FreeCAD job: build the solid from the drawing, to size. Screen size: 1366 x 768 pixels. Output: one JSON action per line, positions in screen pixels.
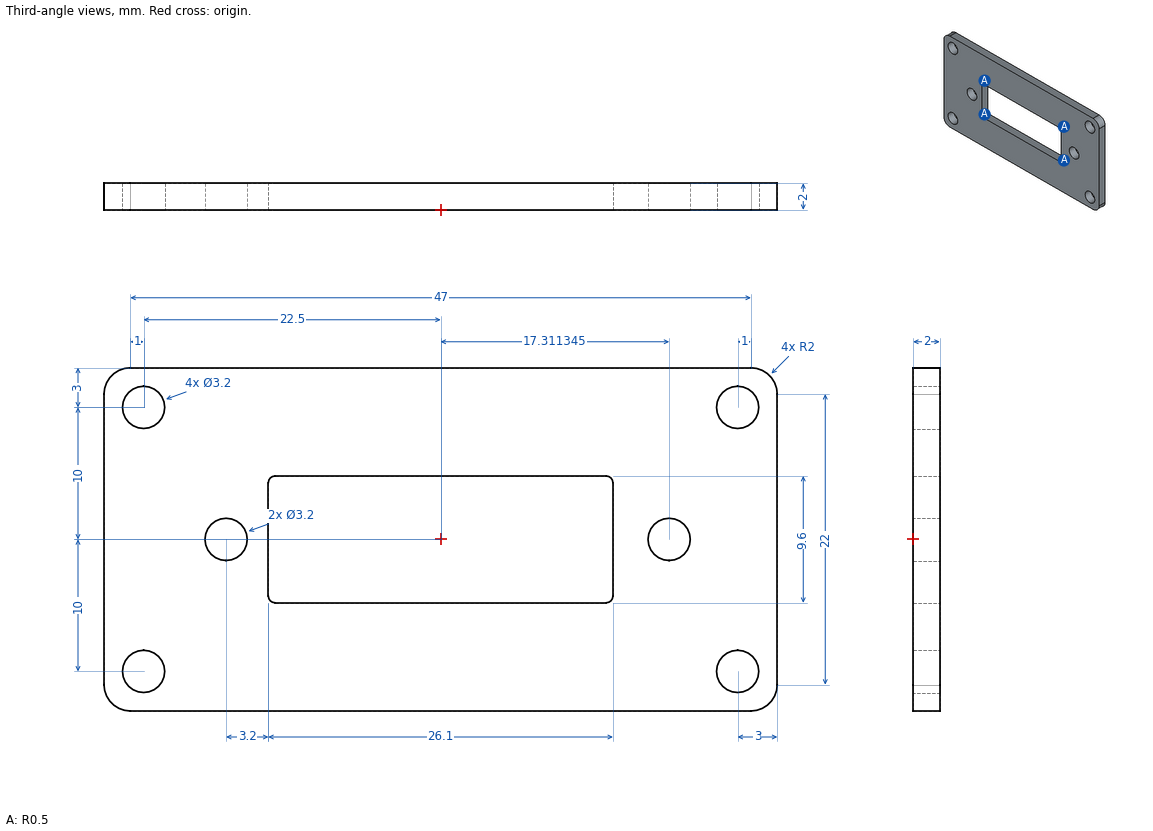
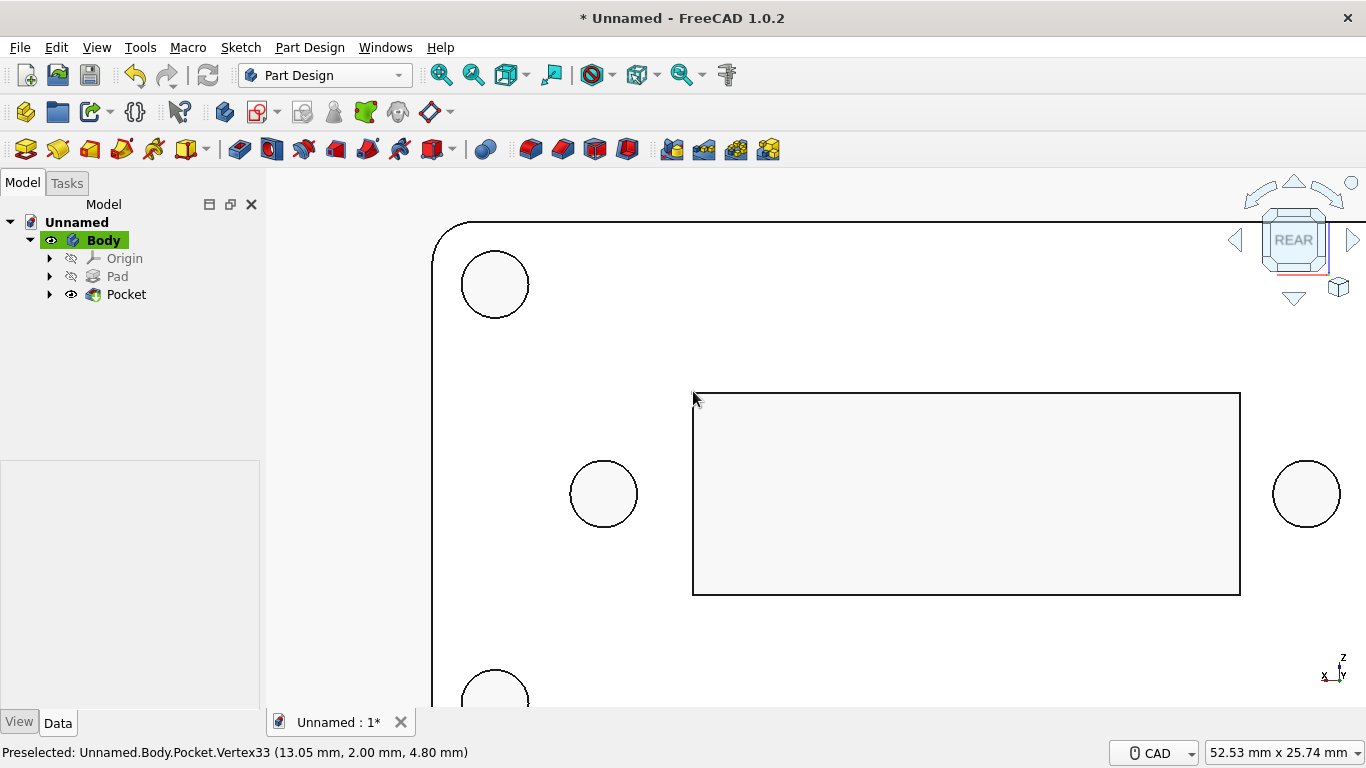
{"action": "left_click", "coordinate": [442, 76]}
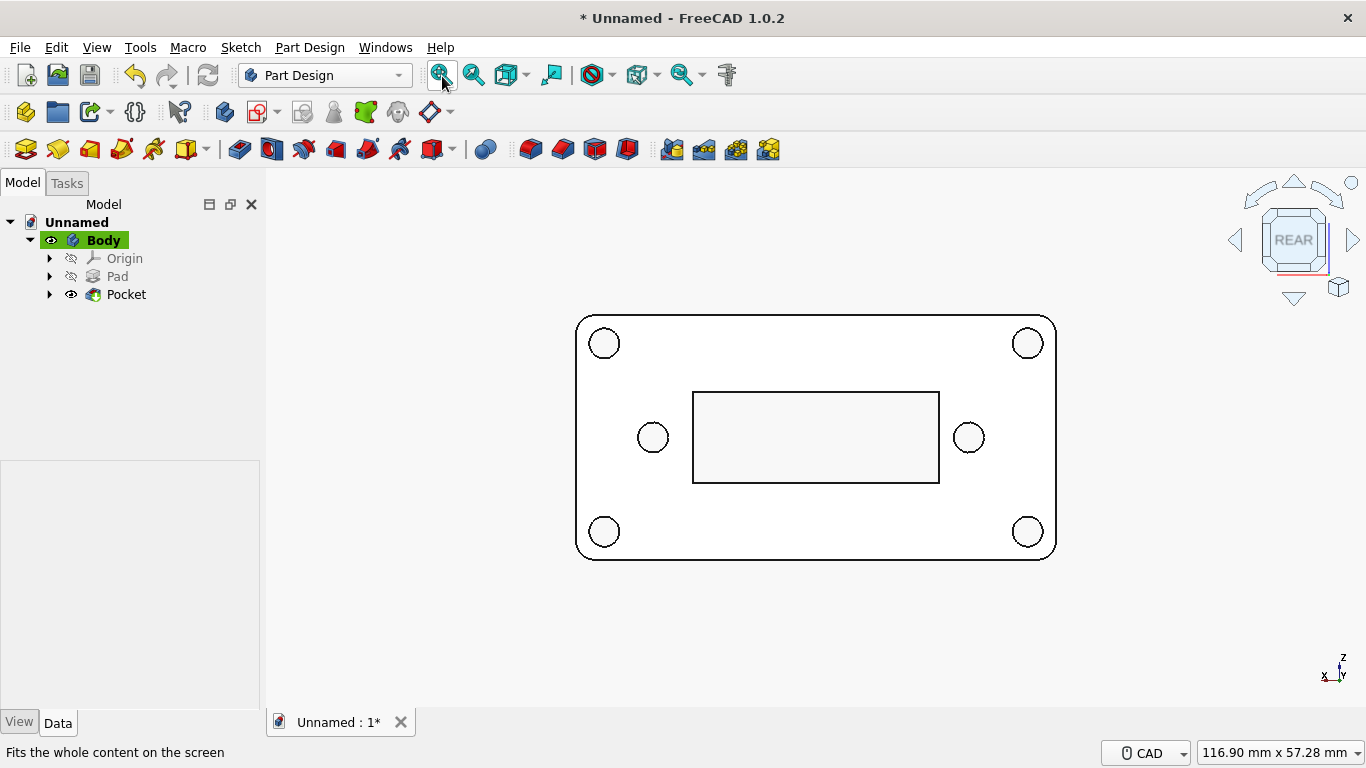
{"action": "key", "text": "6"}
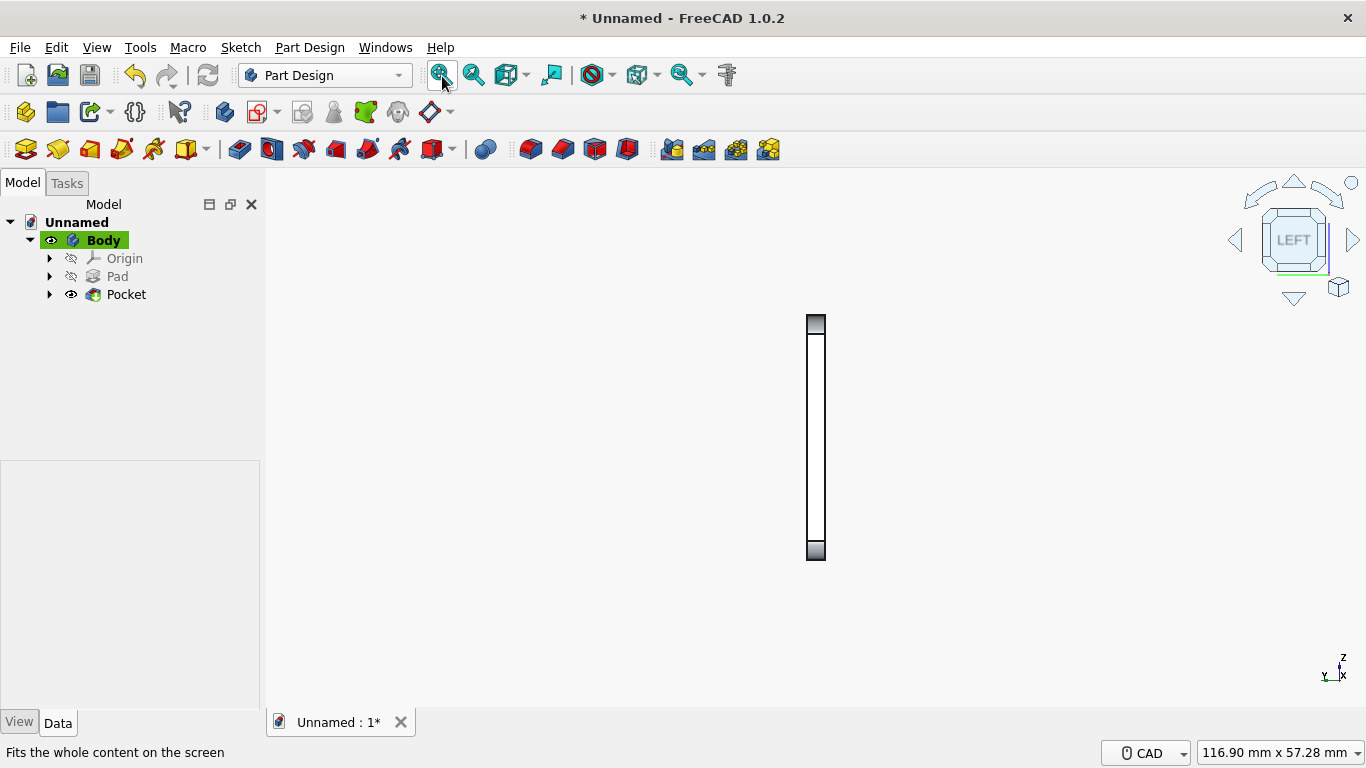
{"action": "scroll", "coordinate": [816, 391], "scroll_direction": "up", "scroll_amount": 4}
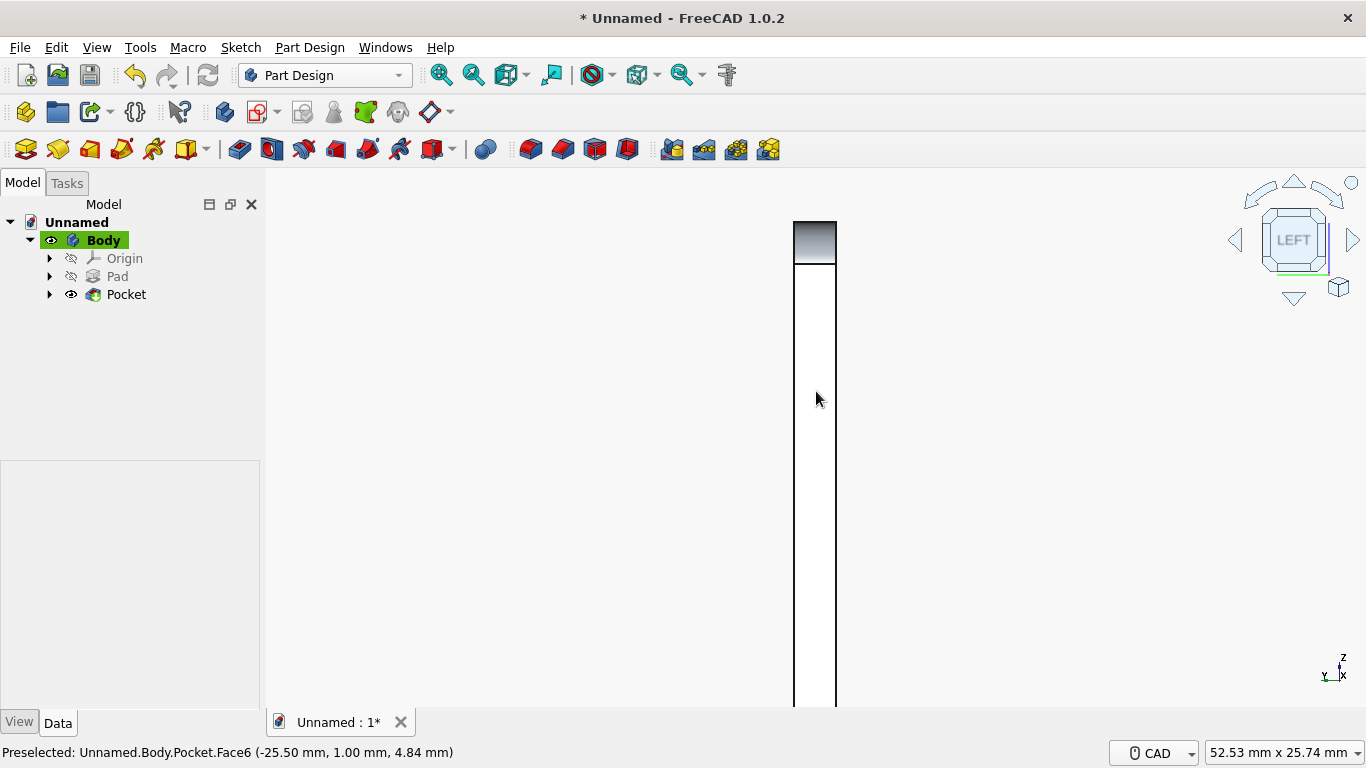
{"action": "left_click", "coordinate": [442, 76]}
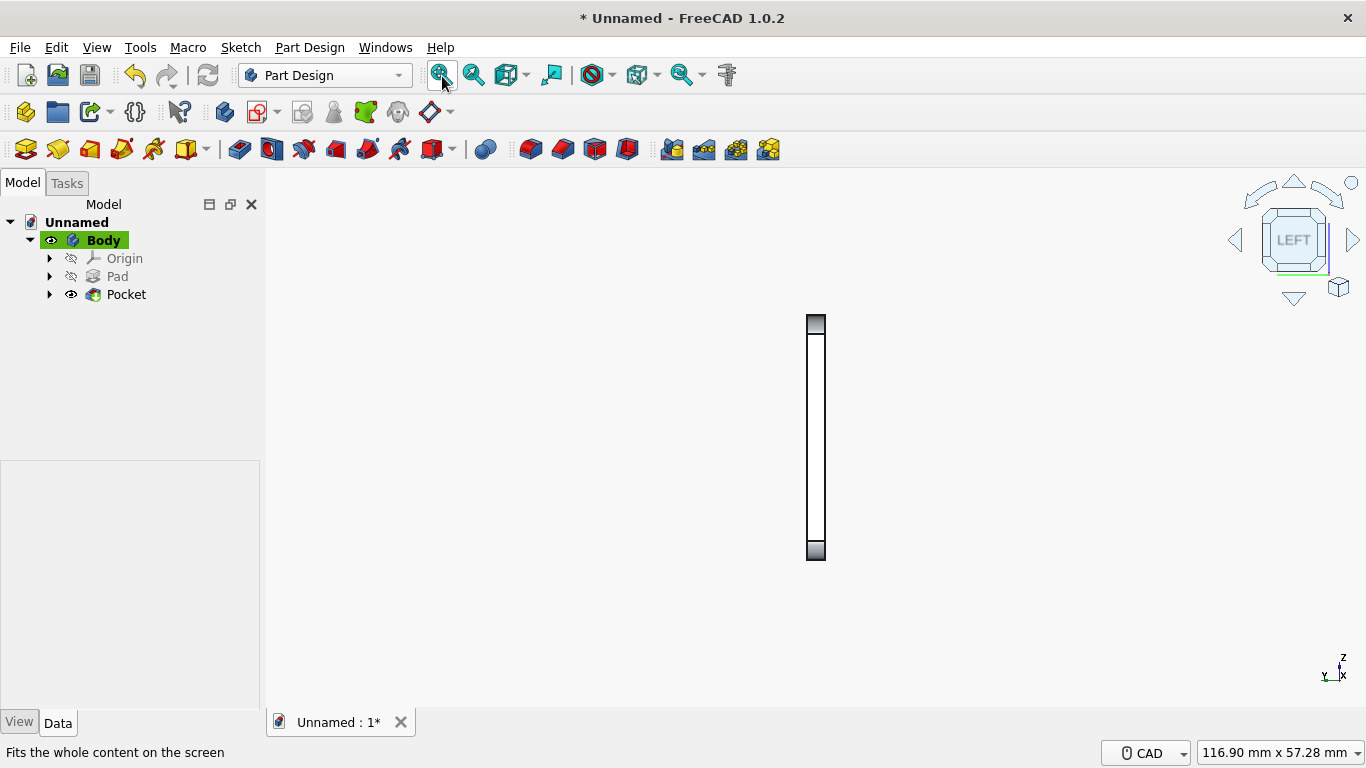
{"action": "key", "text": "v 3"}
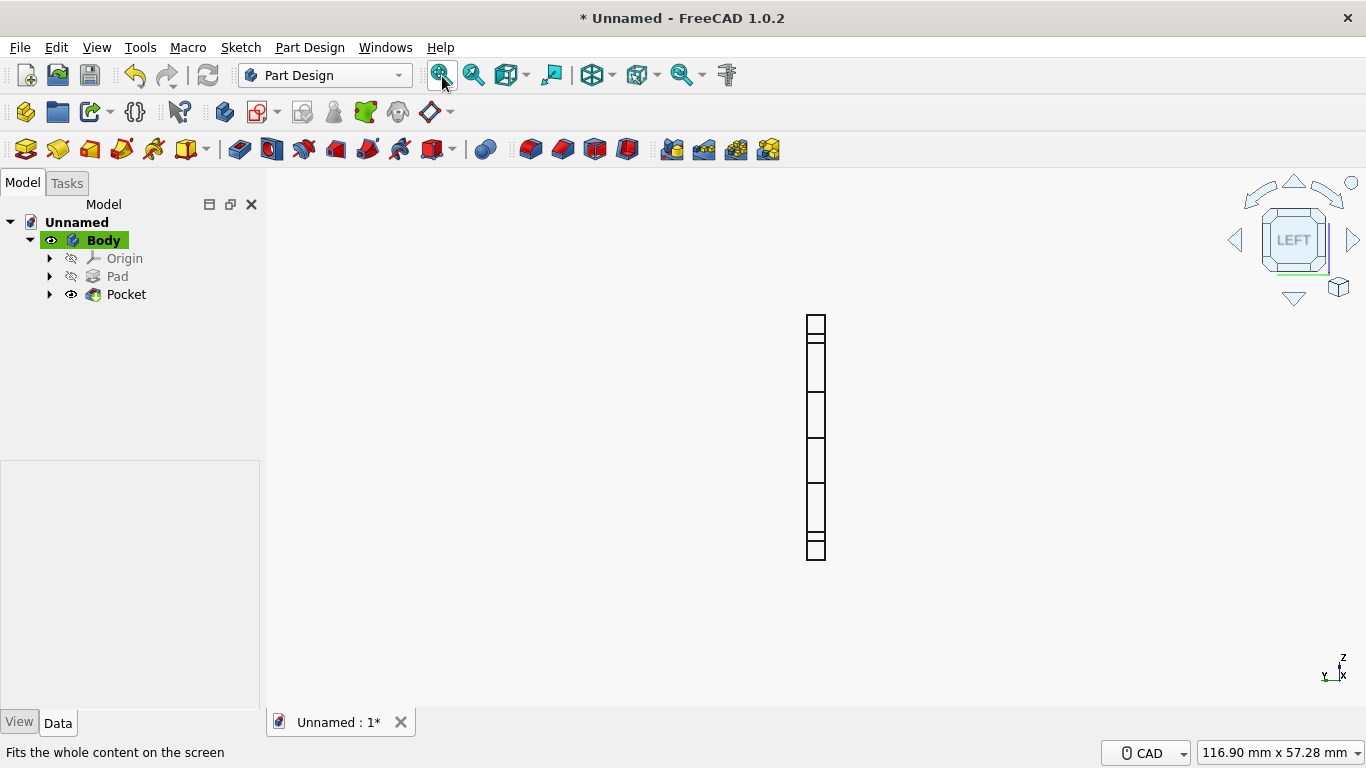
{"action": "key", "text": "0"}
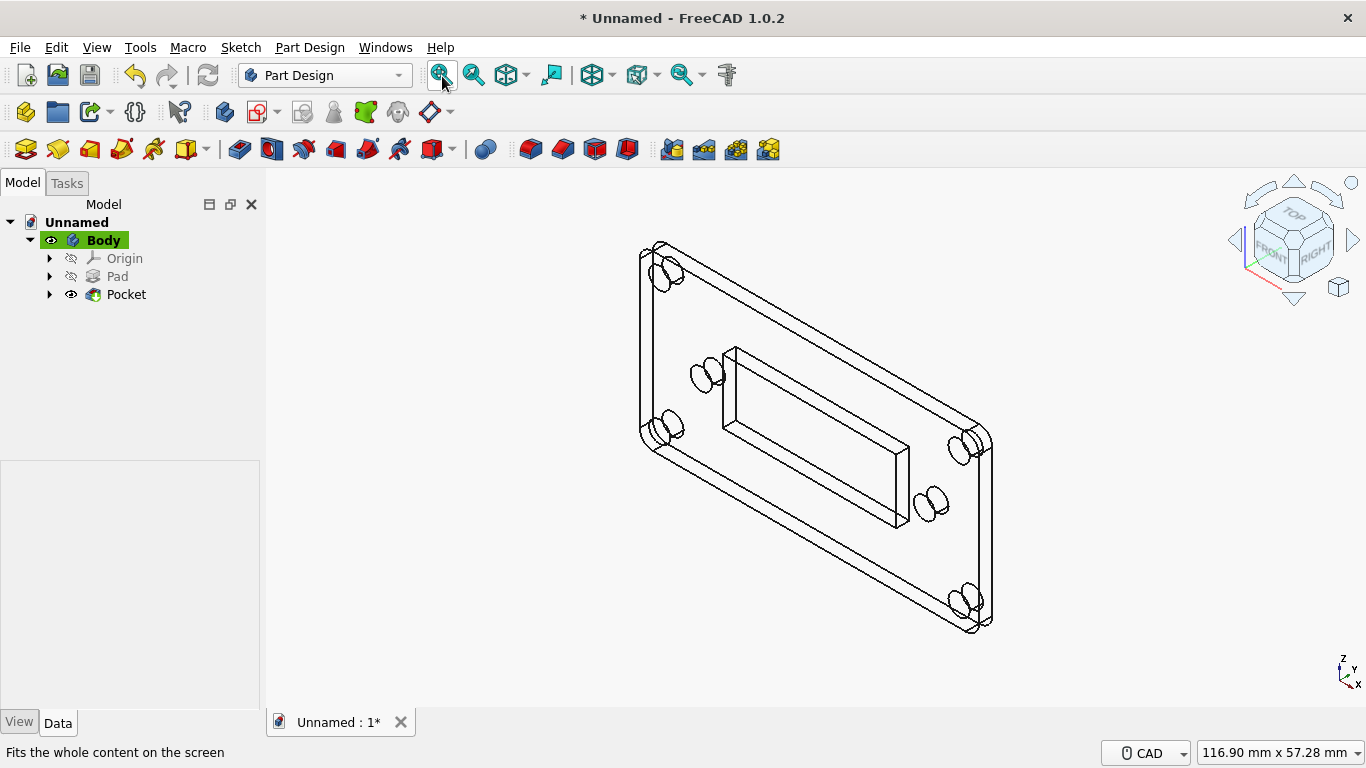
{"action": "left_click", "coordinate": [903, 450]}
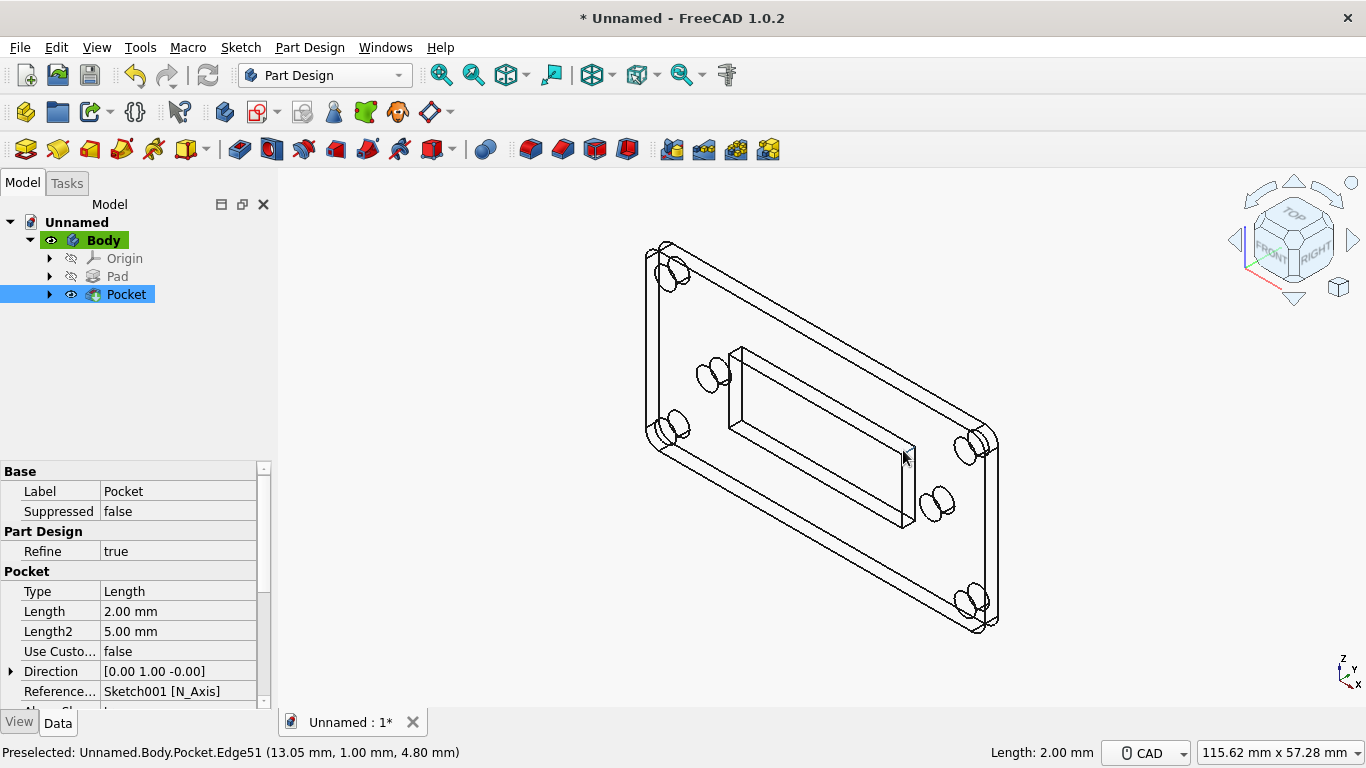
{"action": "left_click", "coordinate": [909, 524], "text": "ctrl"}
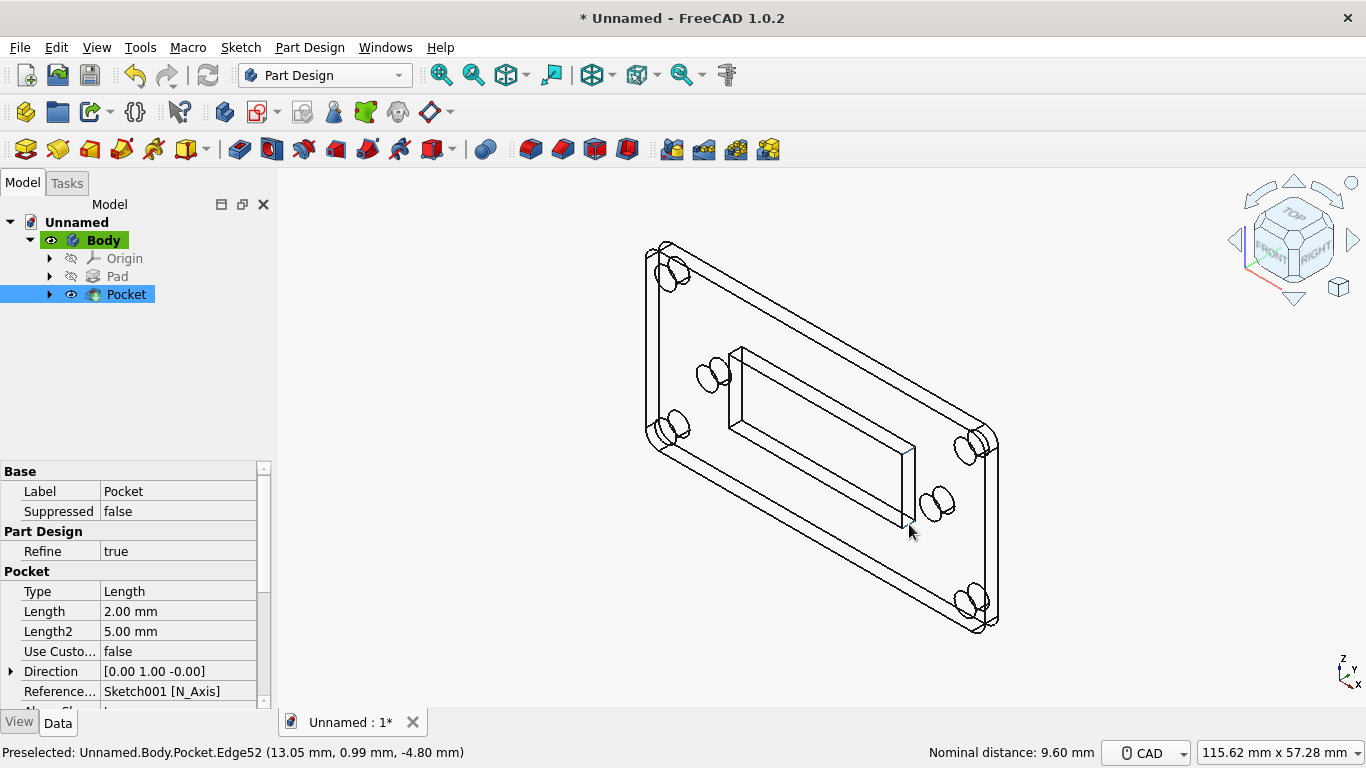
{"action": "left_click", "coordinate": [735, 423], "text": "ctrl"}